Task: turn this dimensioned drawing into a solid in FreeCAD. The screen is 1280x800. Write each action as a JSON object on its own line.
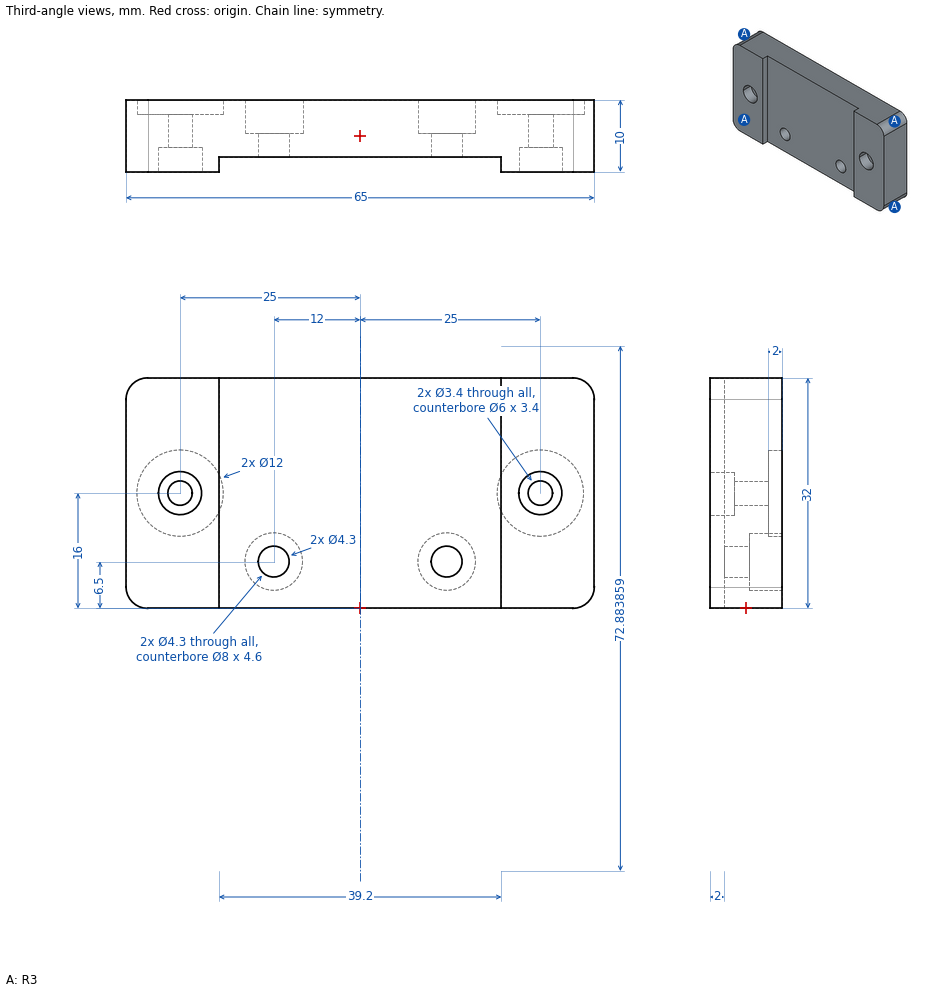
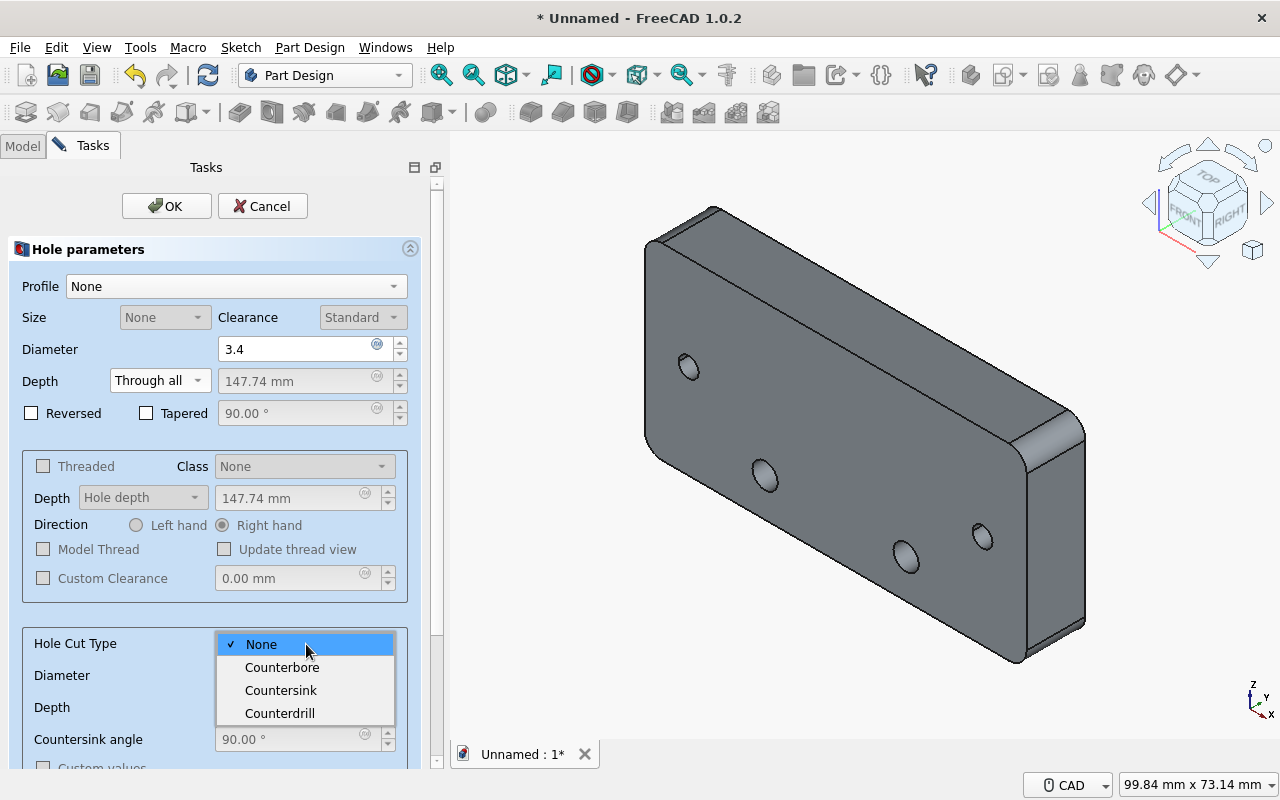
{"action": "left_click", "coordinate": [304, 668]}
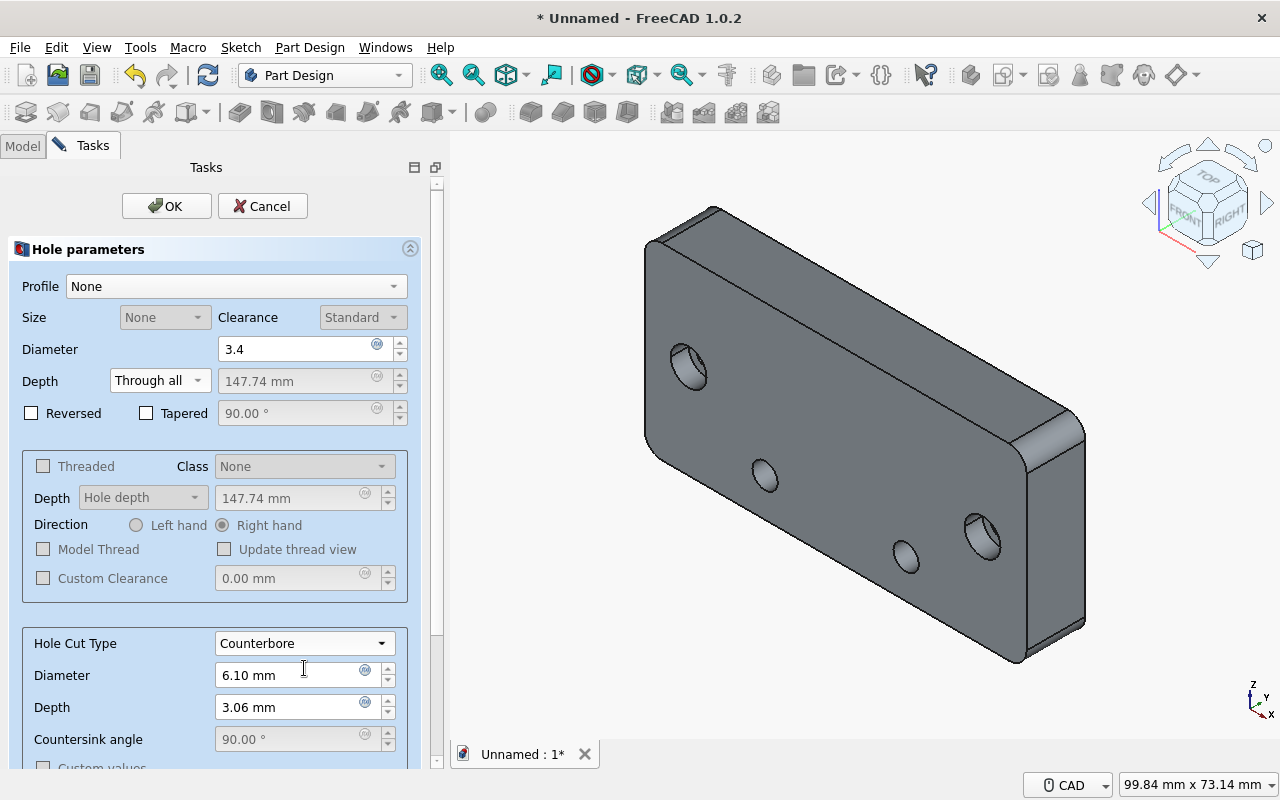
{"action": "triple_click", "coordinate": [298, 675]}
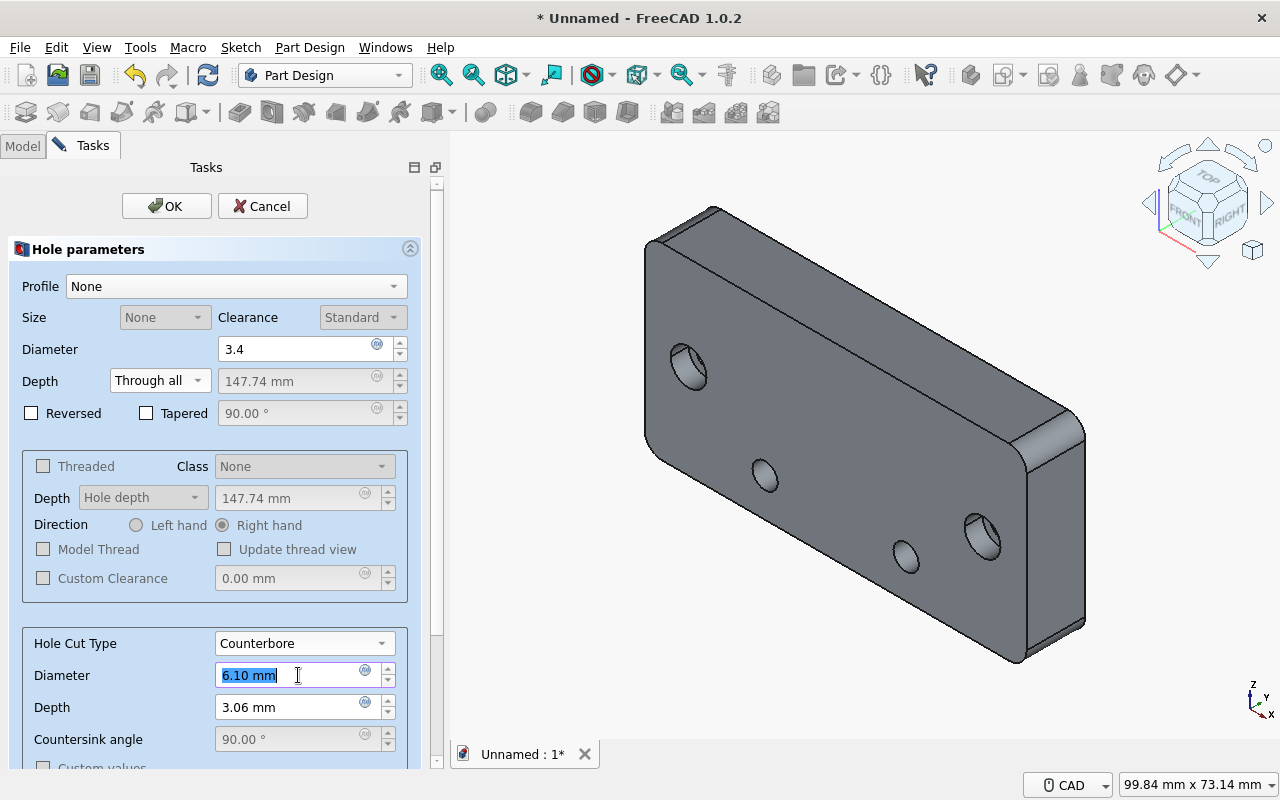
{"action": "type", "text": "6"}
{"action": "key", "text": "Tab"}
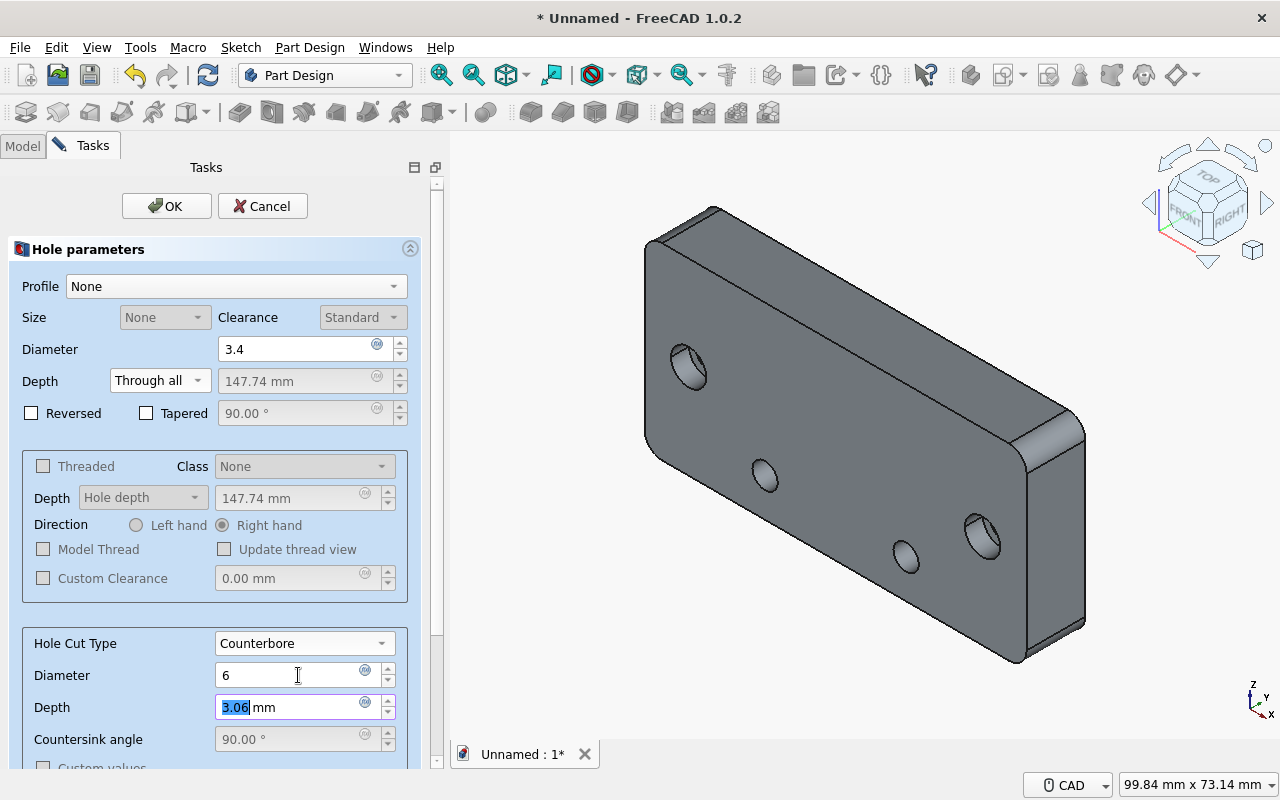
{"action": "type", "text": "3.4"}
{"action": "key", "text": "Tab"}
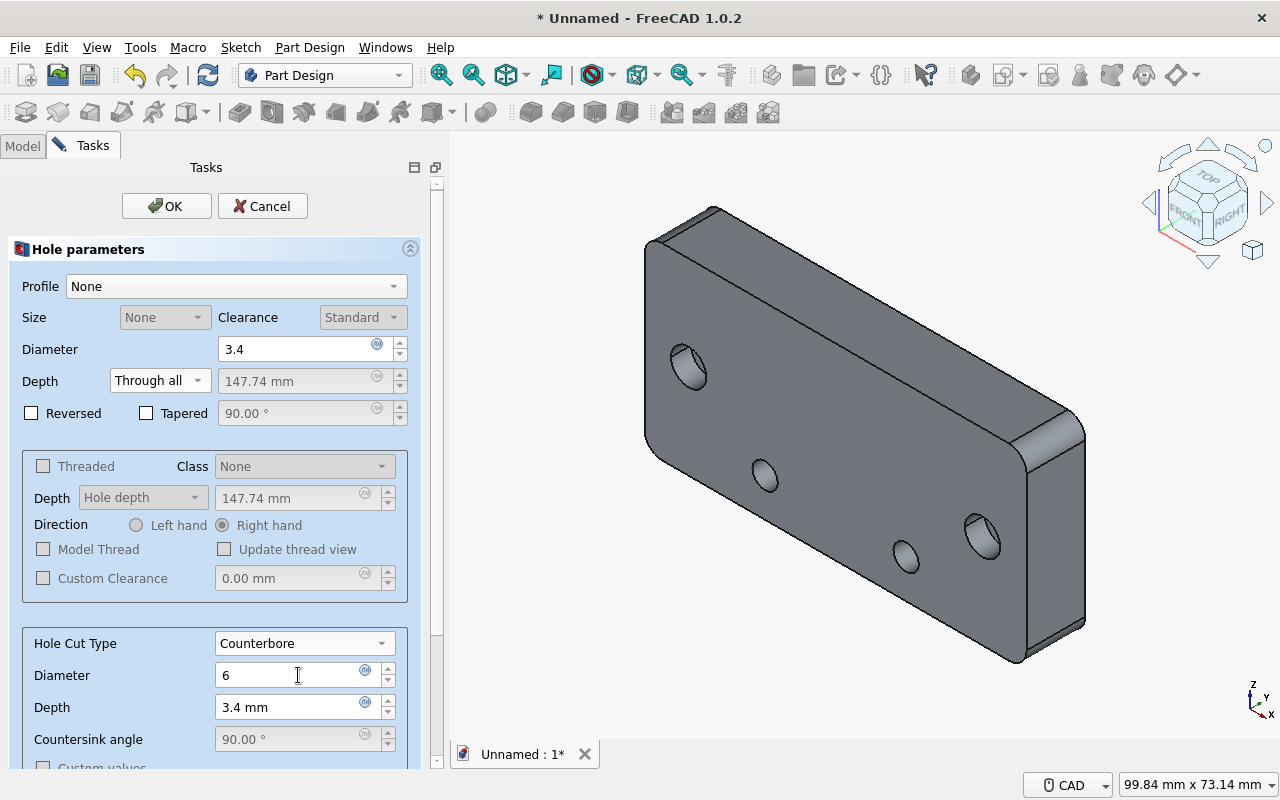
{"action": "left_click", "coordinate": [167, 206]}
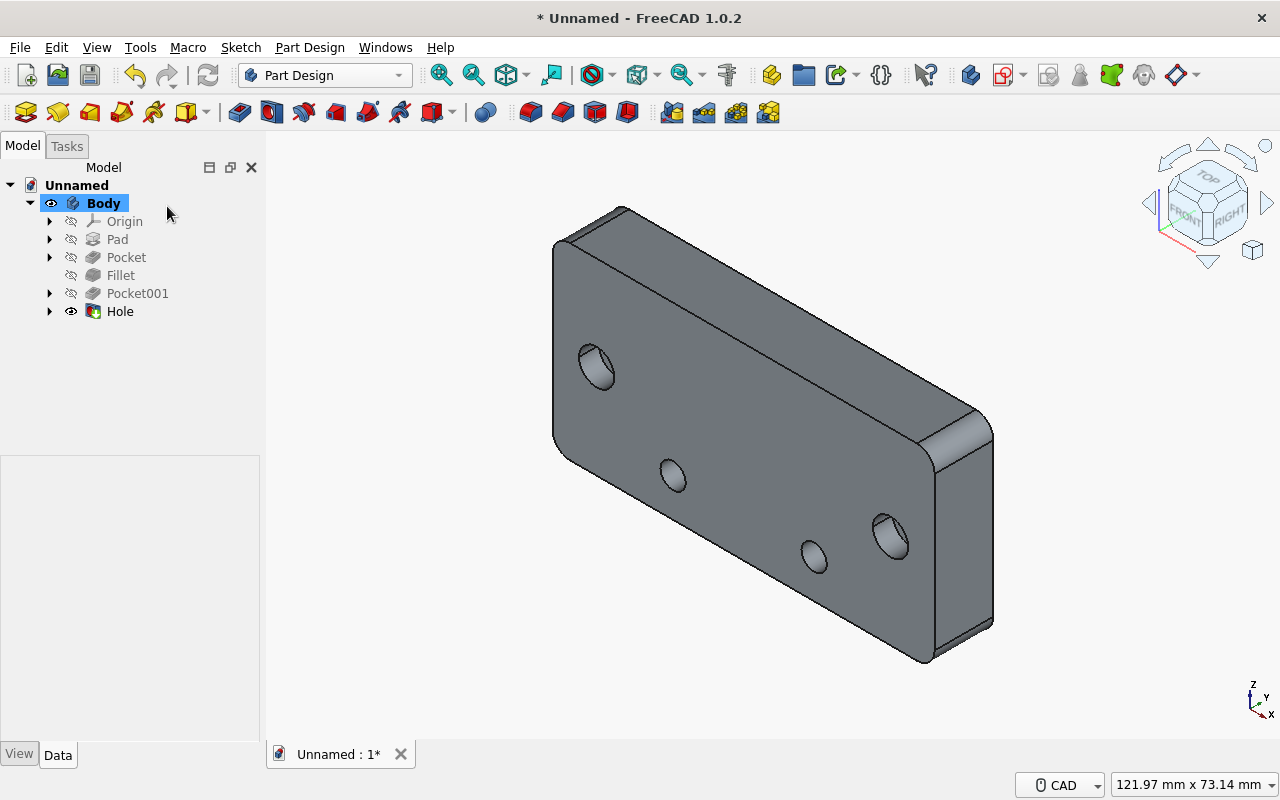
{"action": "key", "text": "4"}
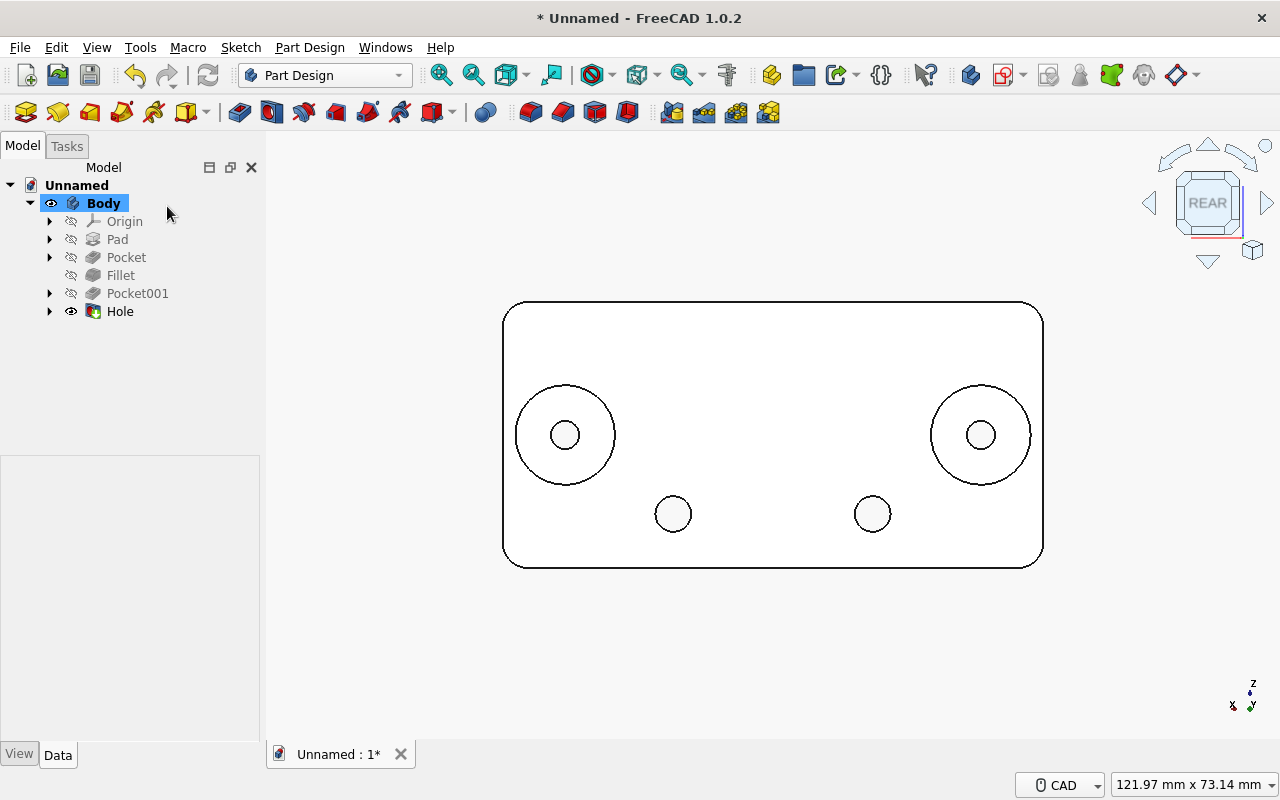
{"action": "left_click", "coordinate": [773, 434]}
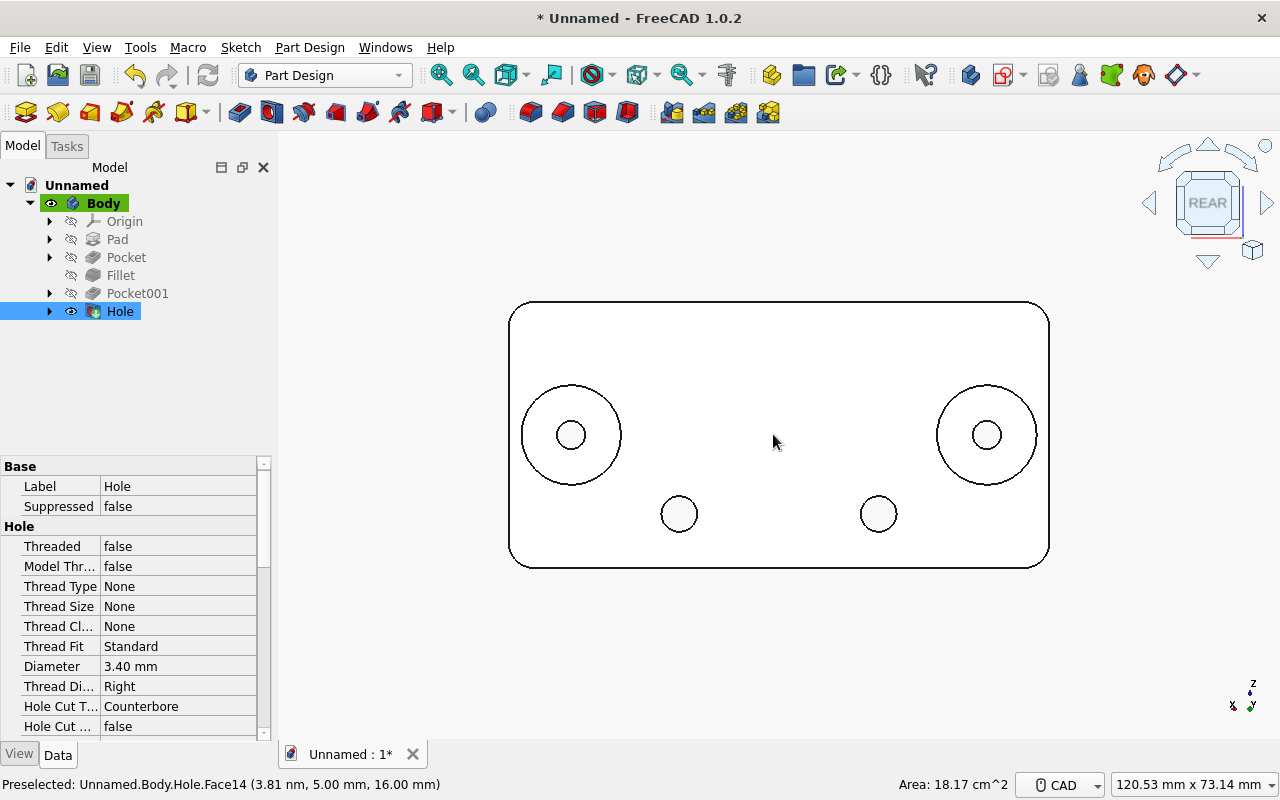
{"action": "left_click", "coordinate": [1004, 76]}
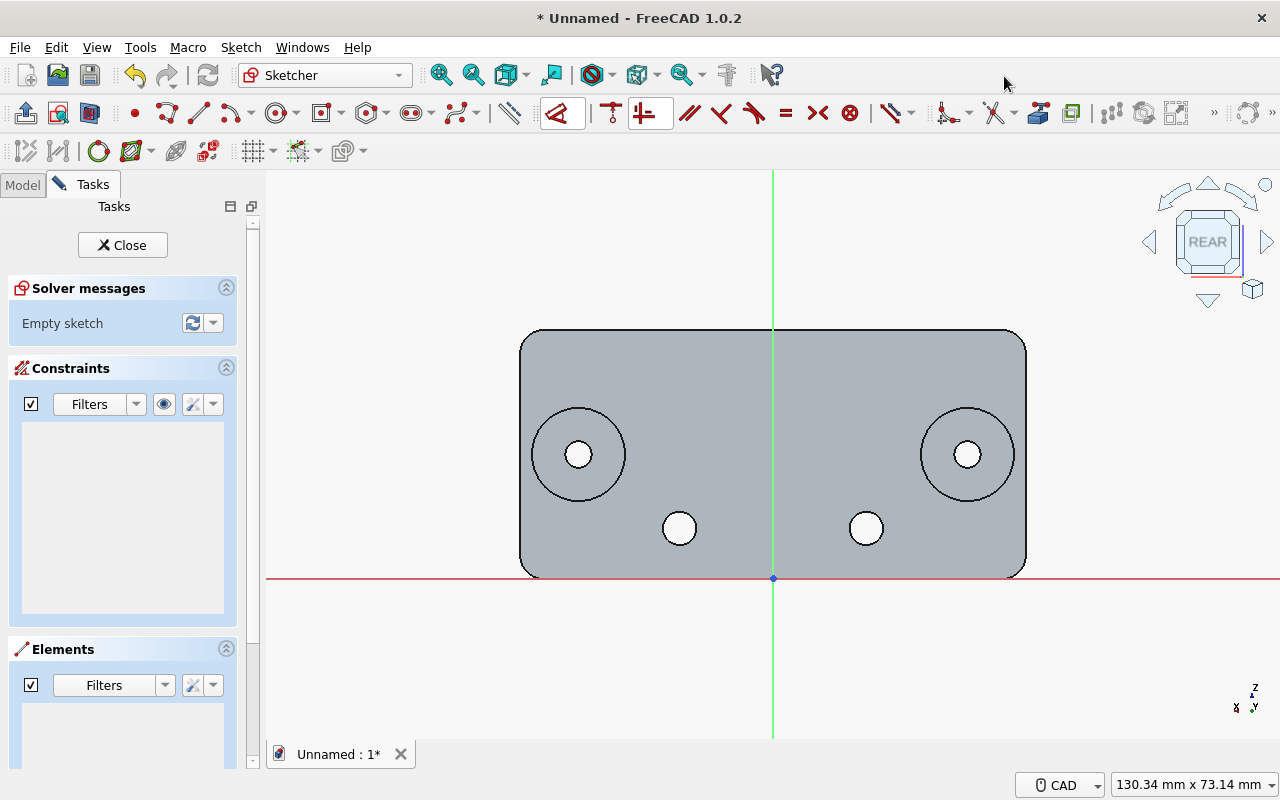
{"action": "scroll", "coordinate": [813, 598], "scroll_direction": "up", "scroll_amount": 5}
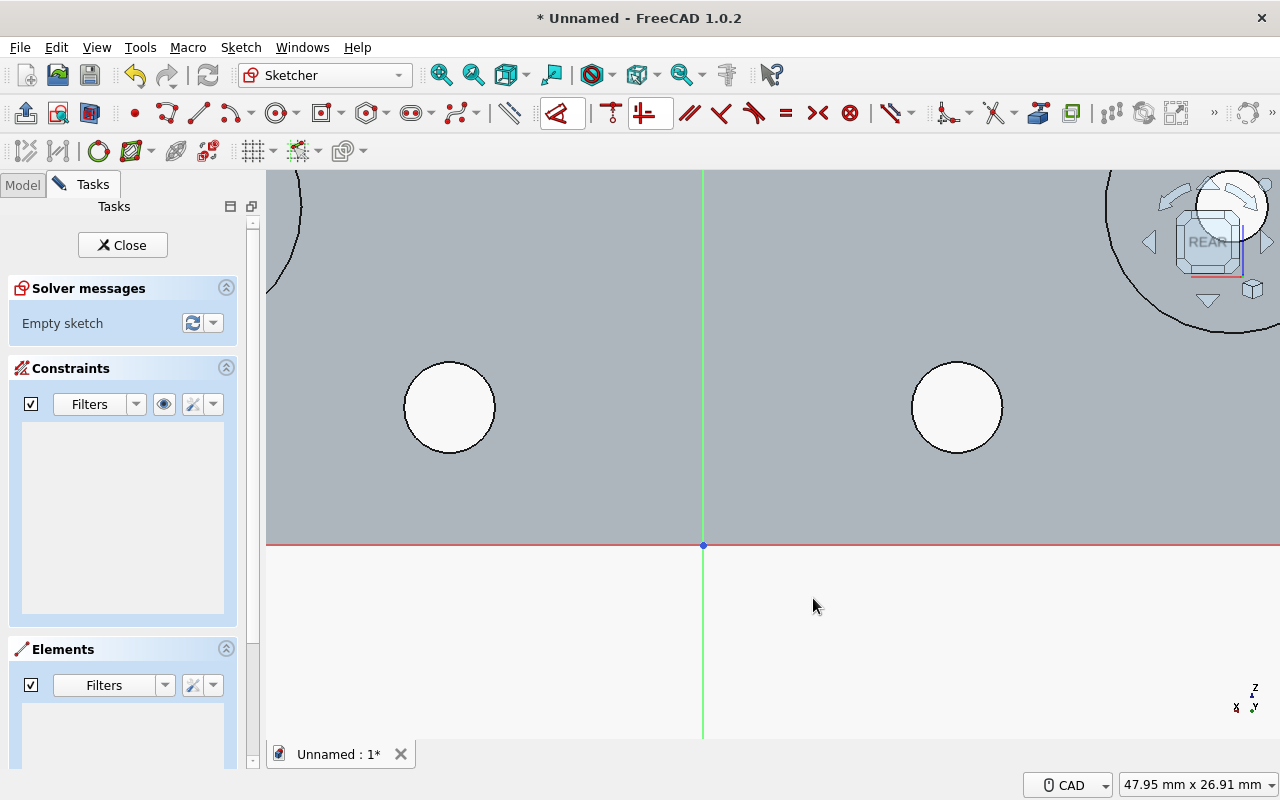
{"action": "left_click", "coordinate": [276, 114]}